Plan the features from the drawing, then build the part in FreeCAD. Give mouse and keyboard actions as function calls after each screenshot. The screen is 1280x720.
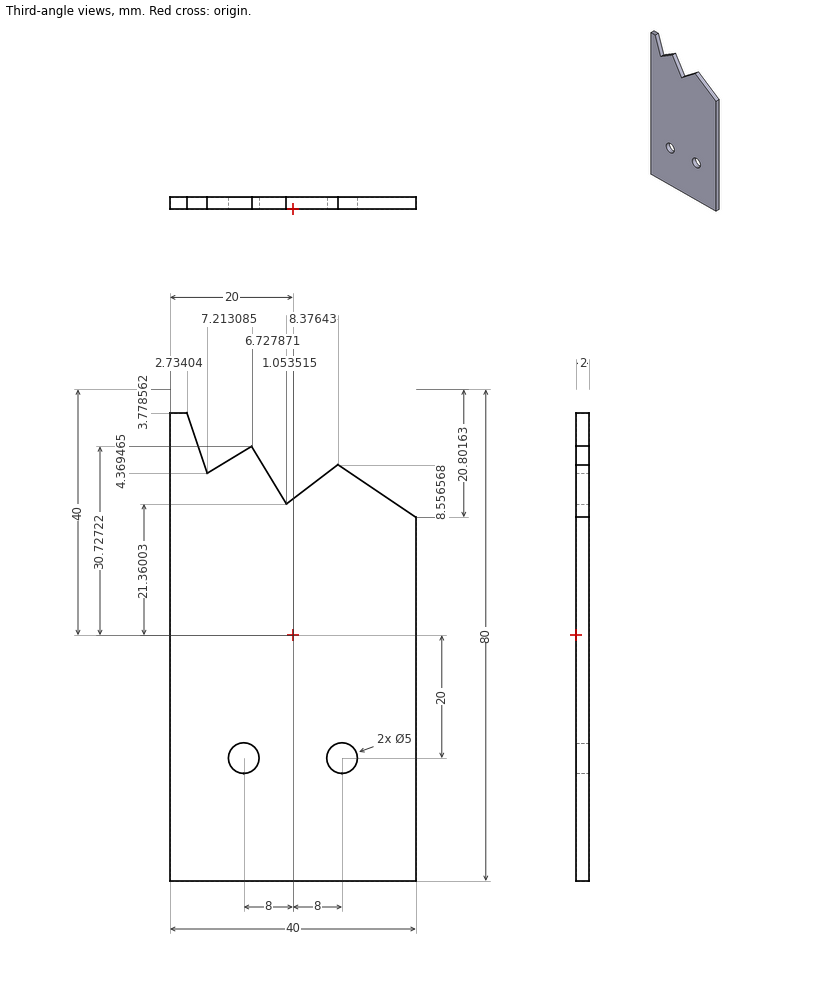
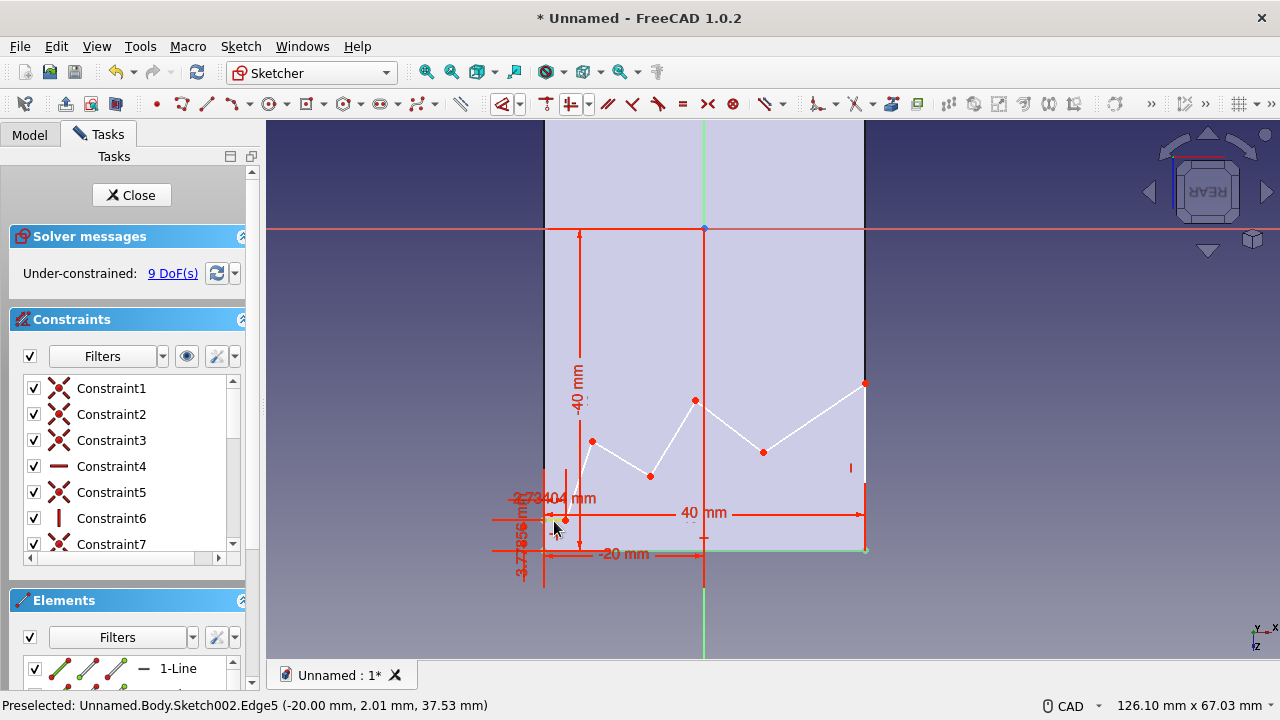
click(865, 501)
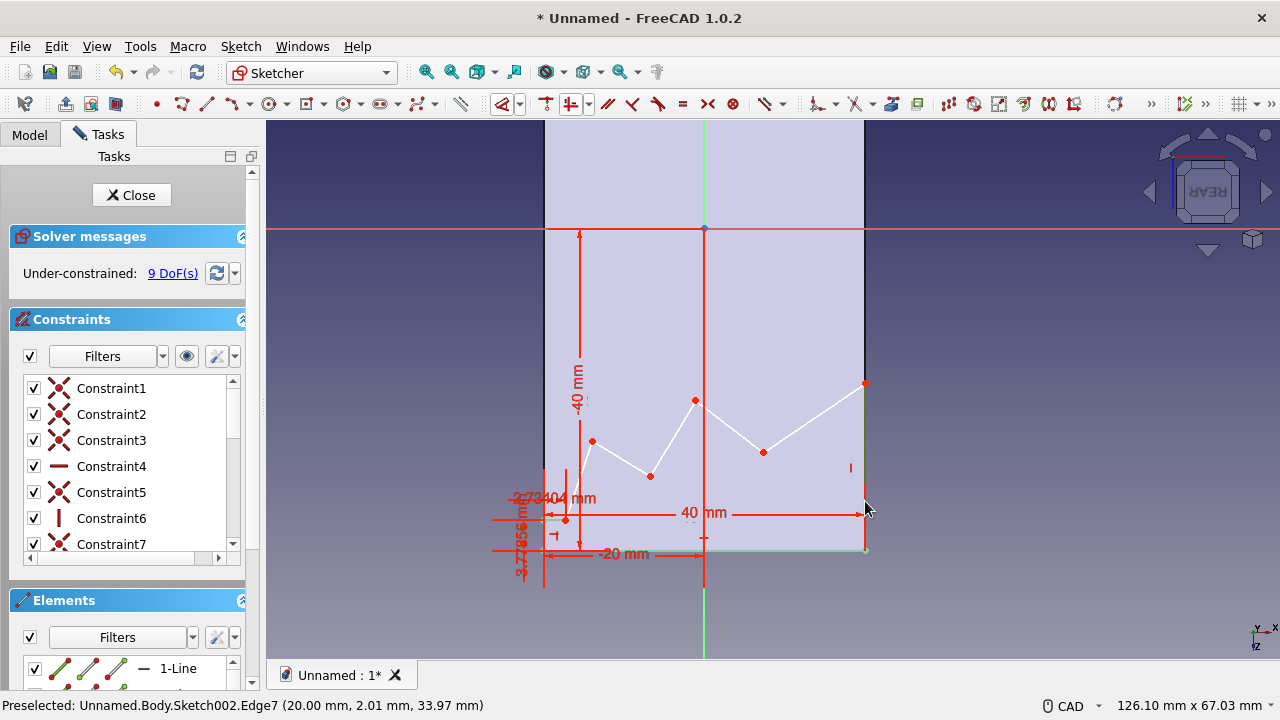
key(i)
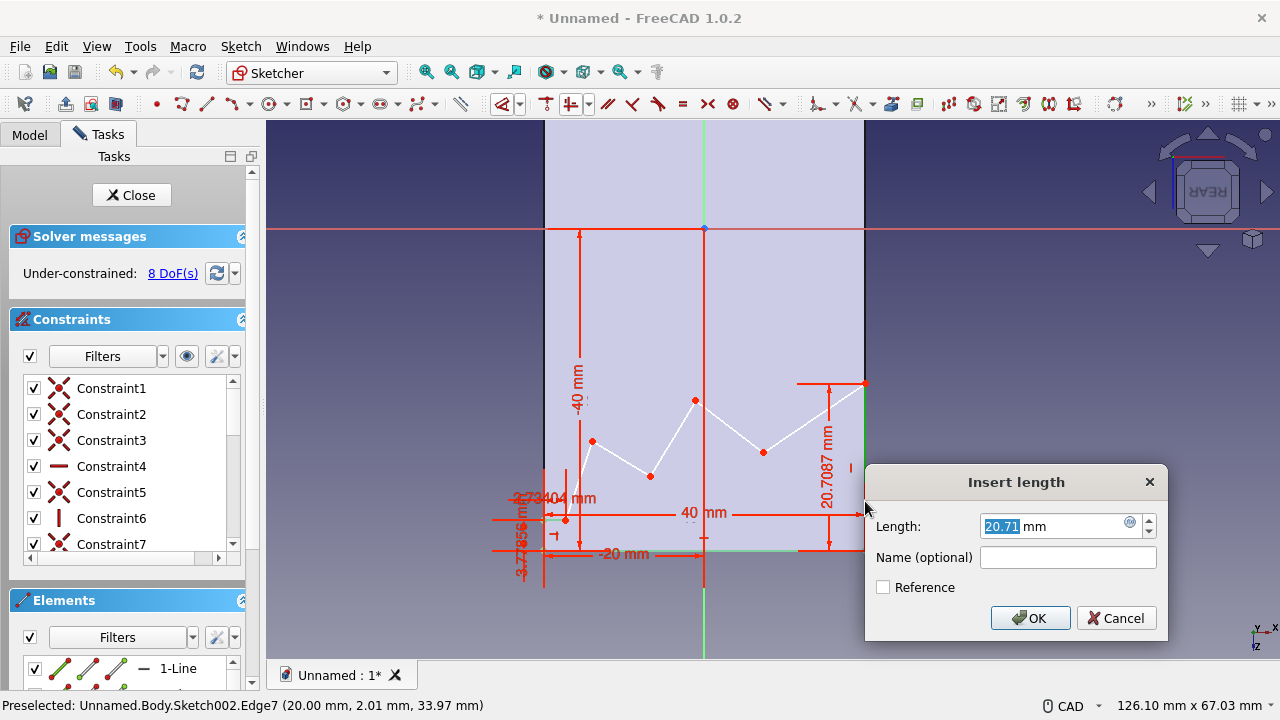
text(20.80163)
key(Return)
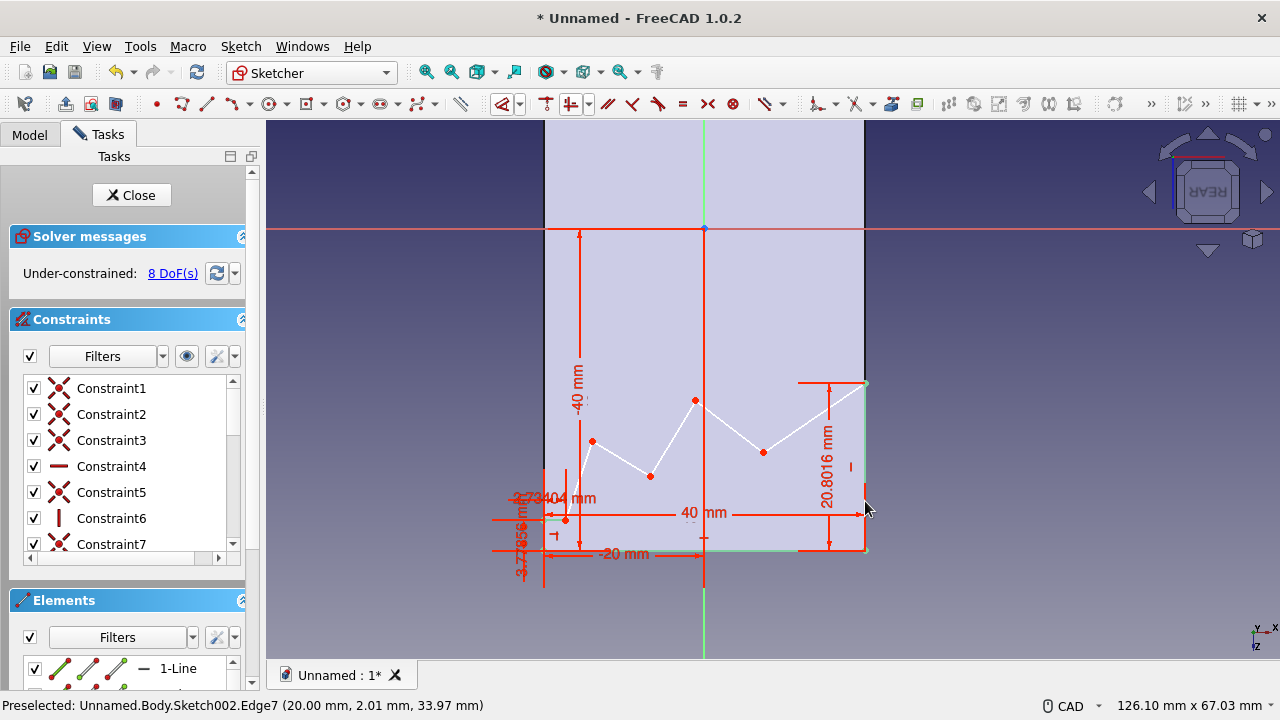
click(743, 437)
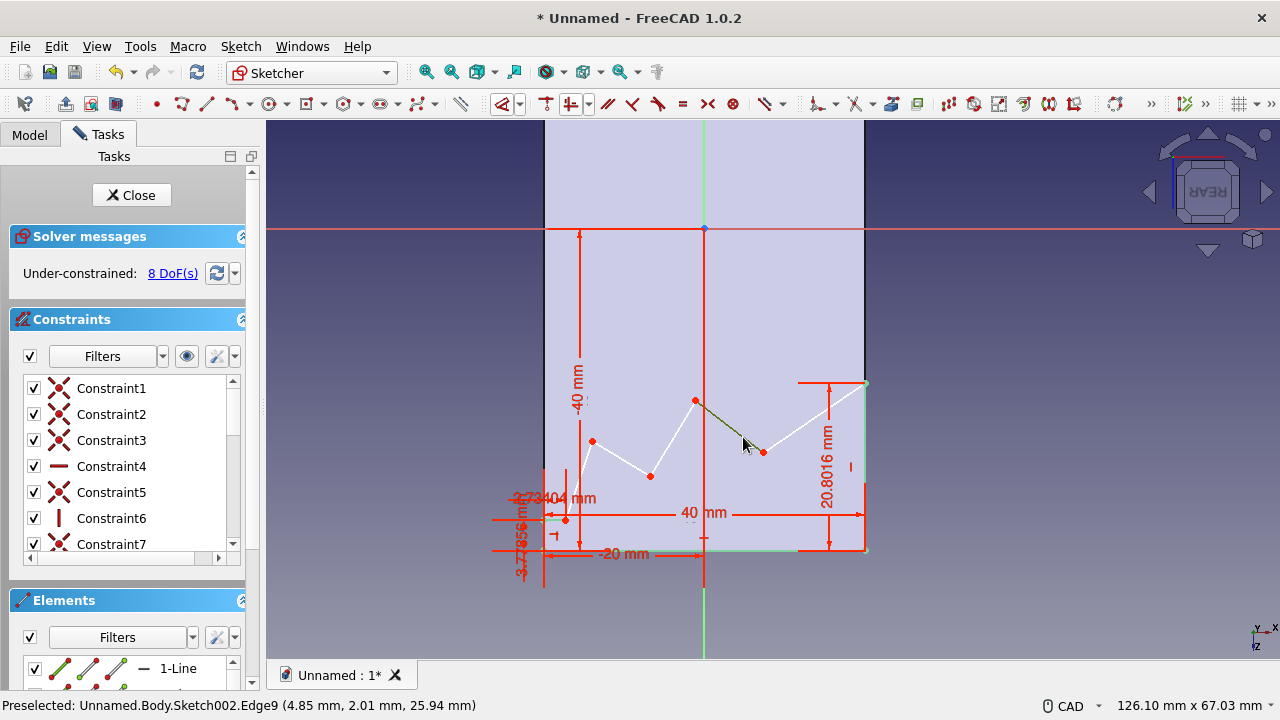
key(l)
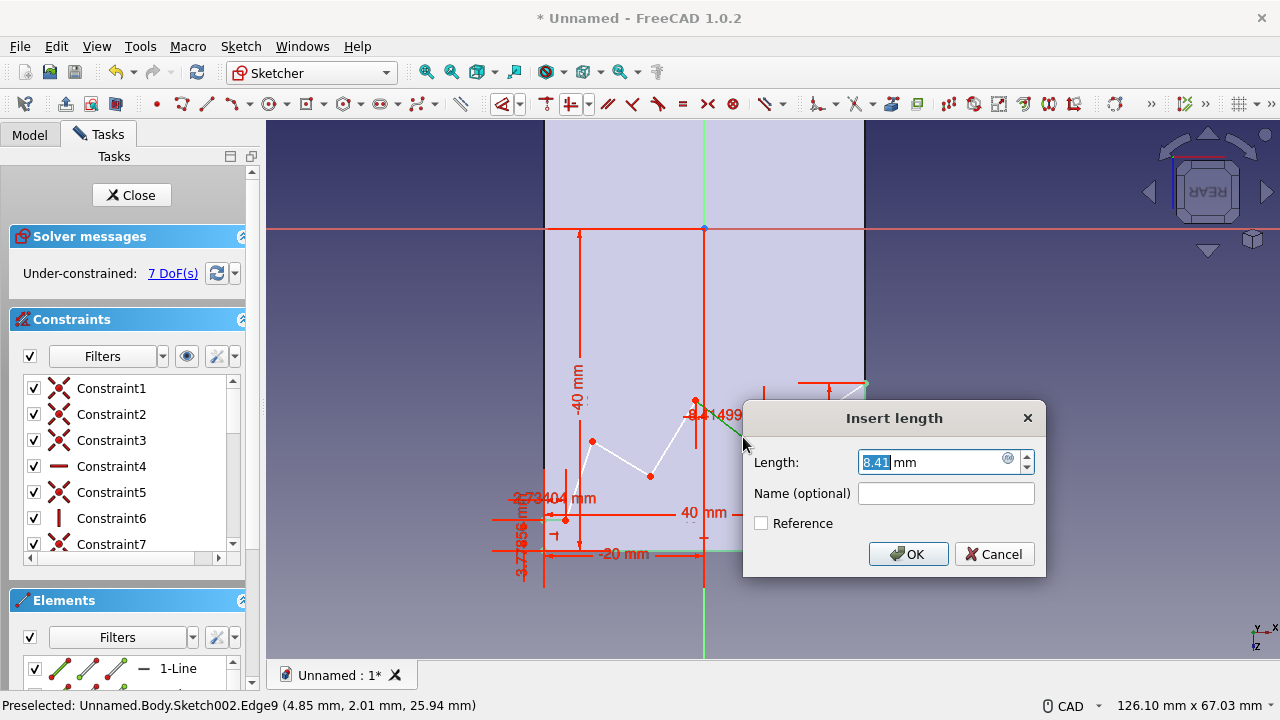
text(8.37643)
key(Return)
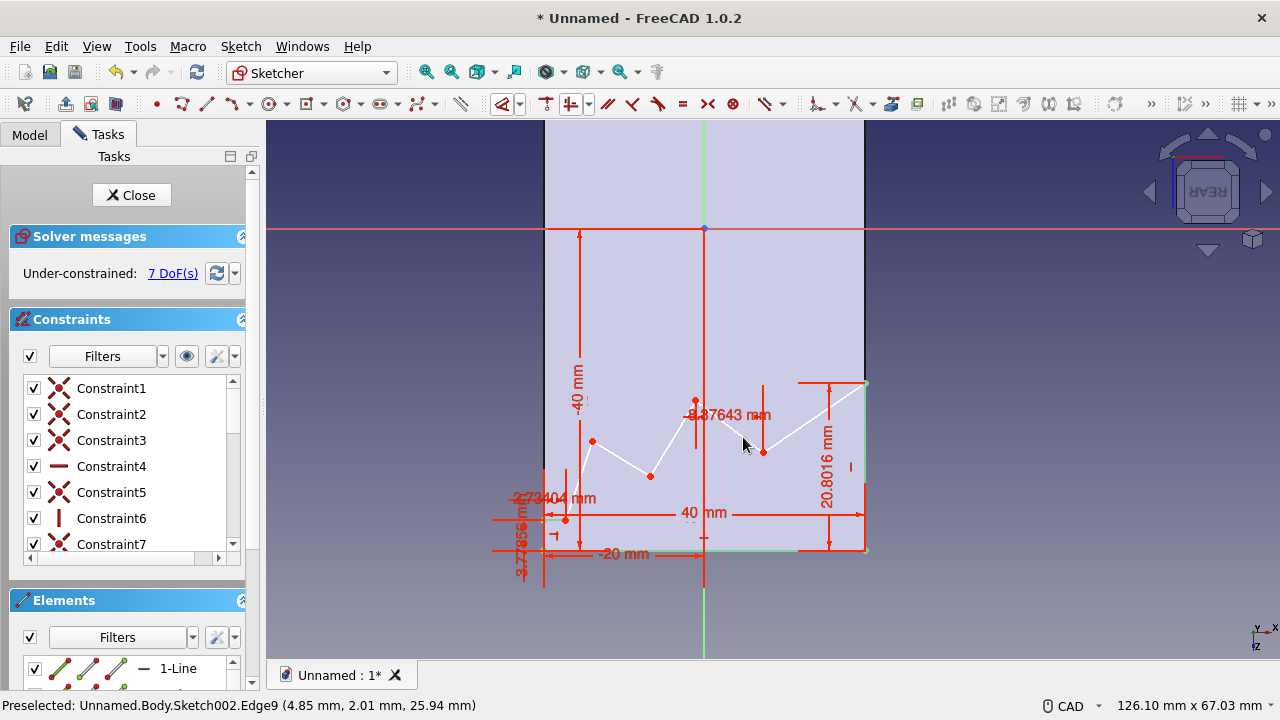
scroll(696, 401, up, 8)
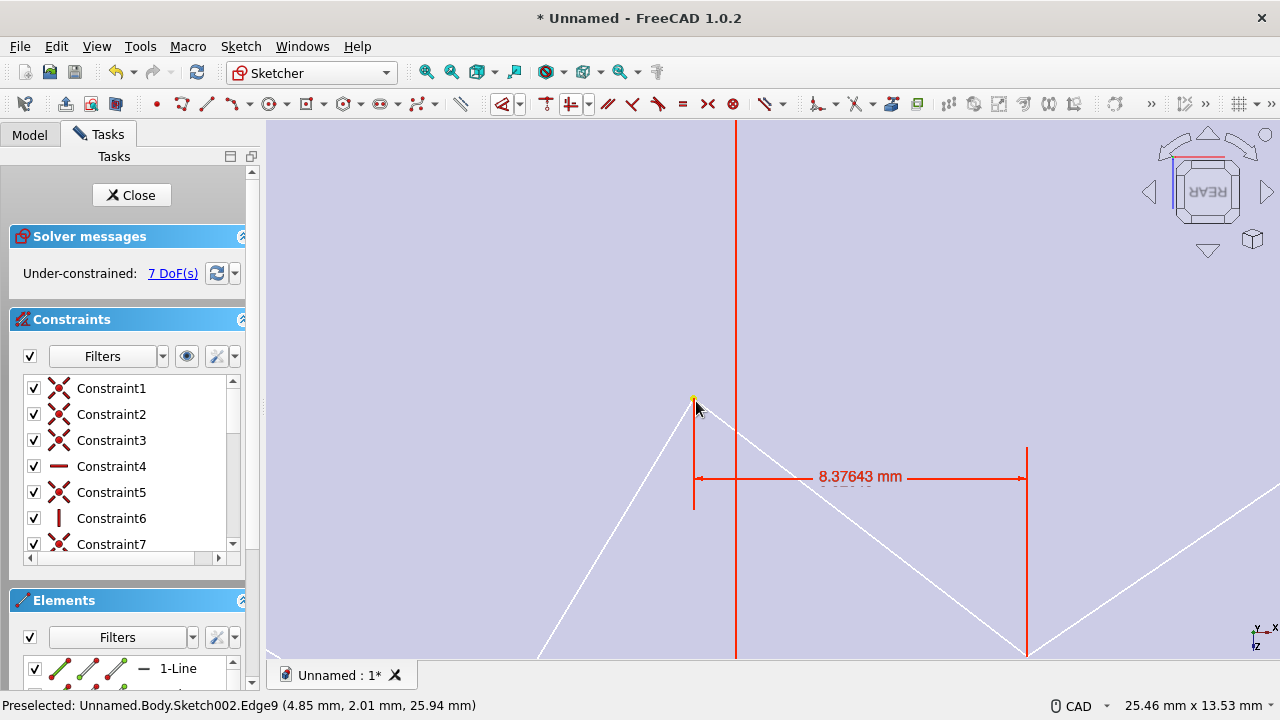
click(694, 399)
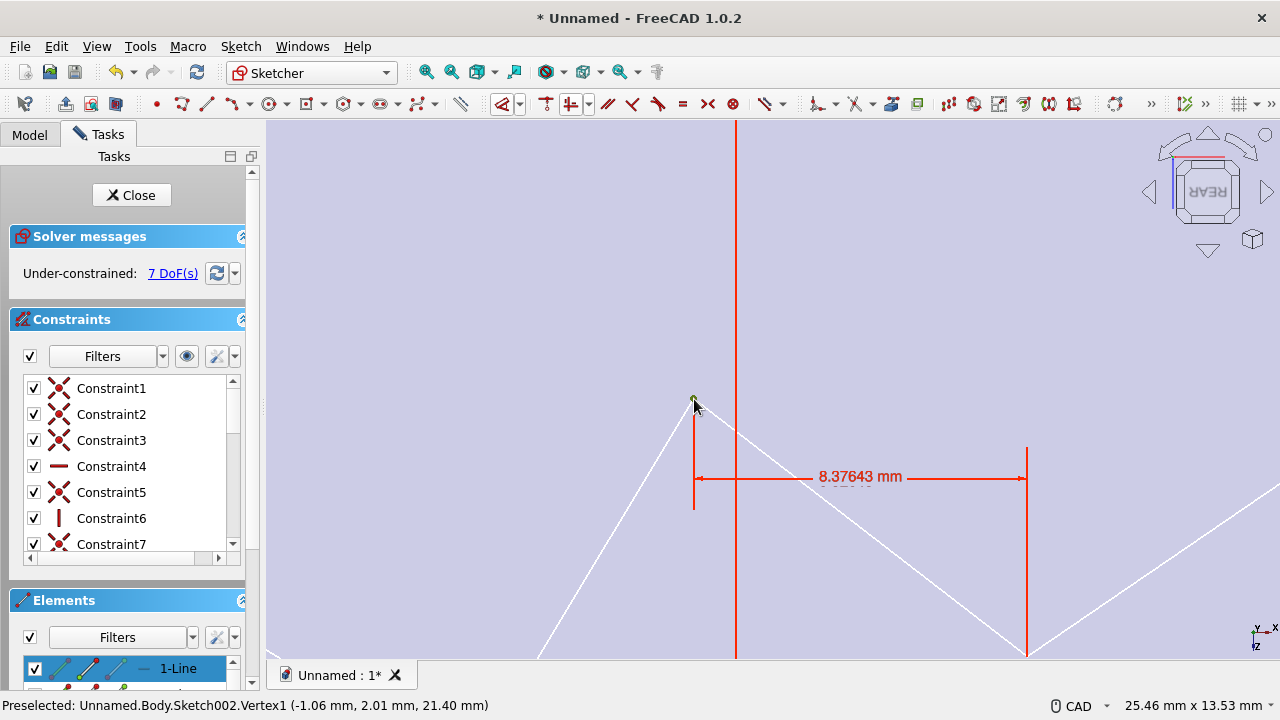
key(l)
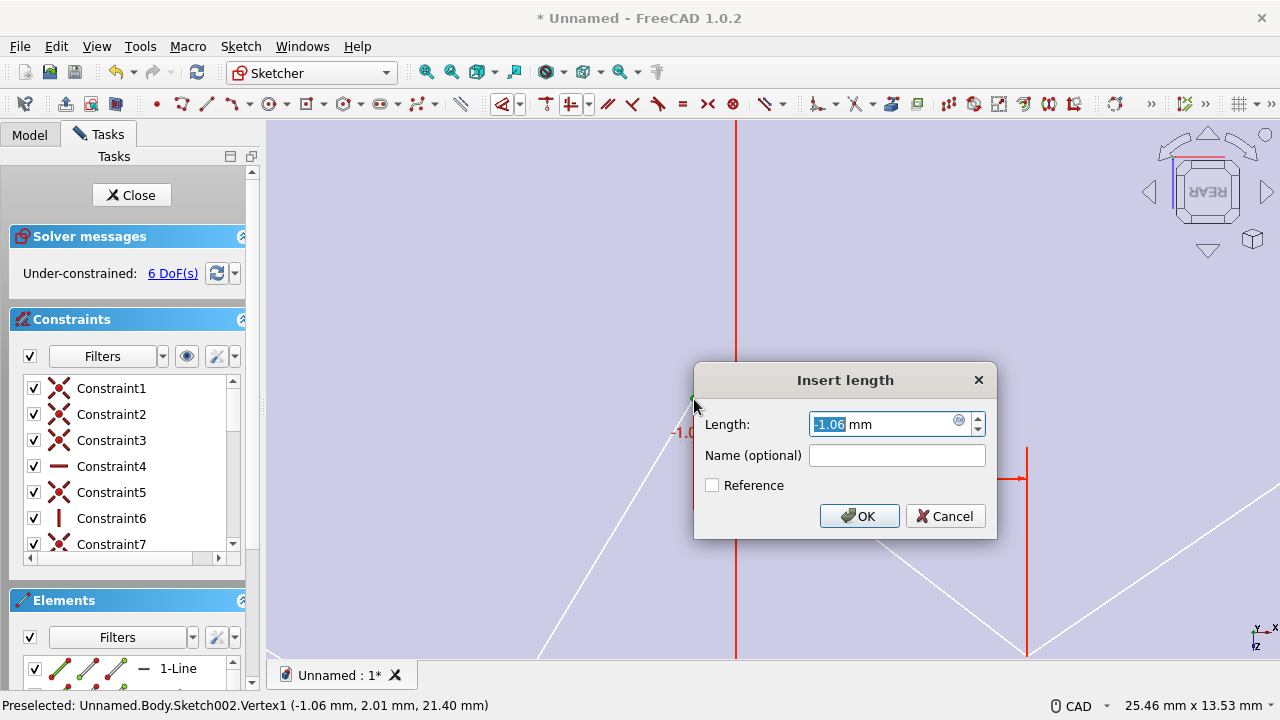
text(-1.053515)
key(Return)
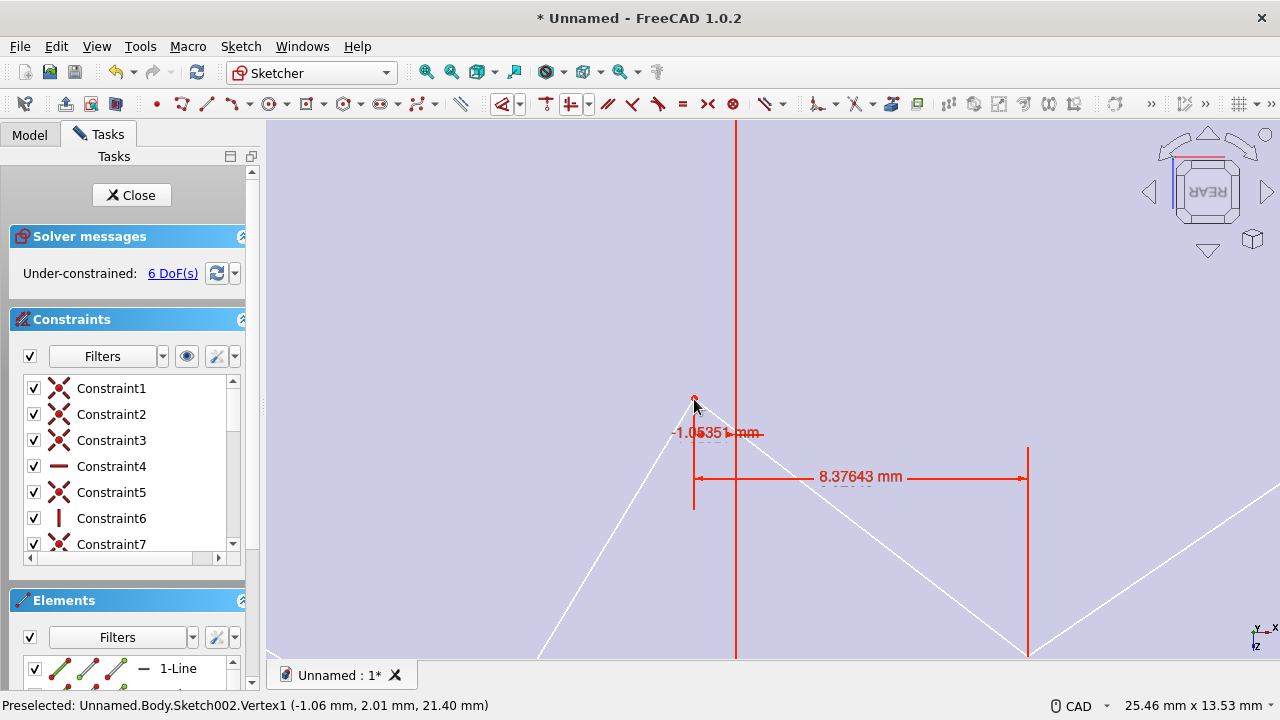
scroll(697, 401, down, 8)